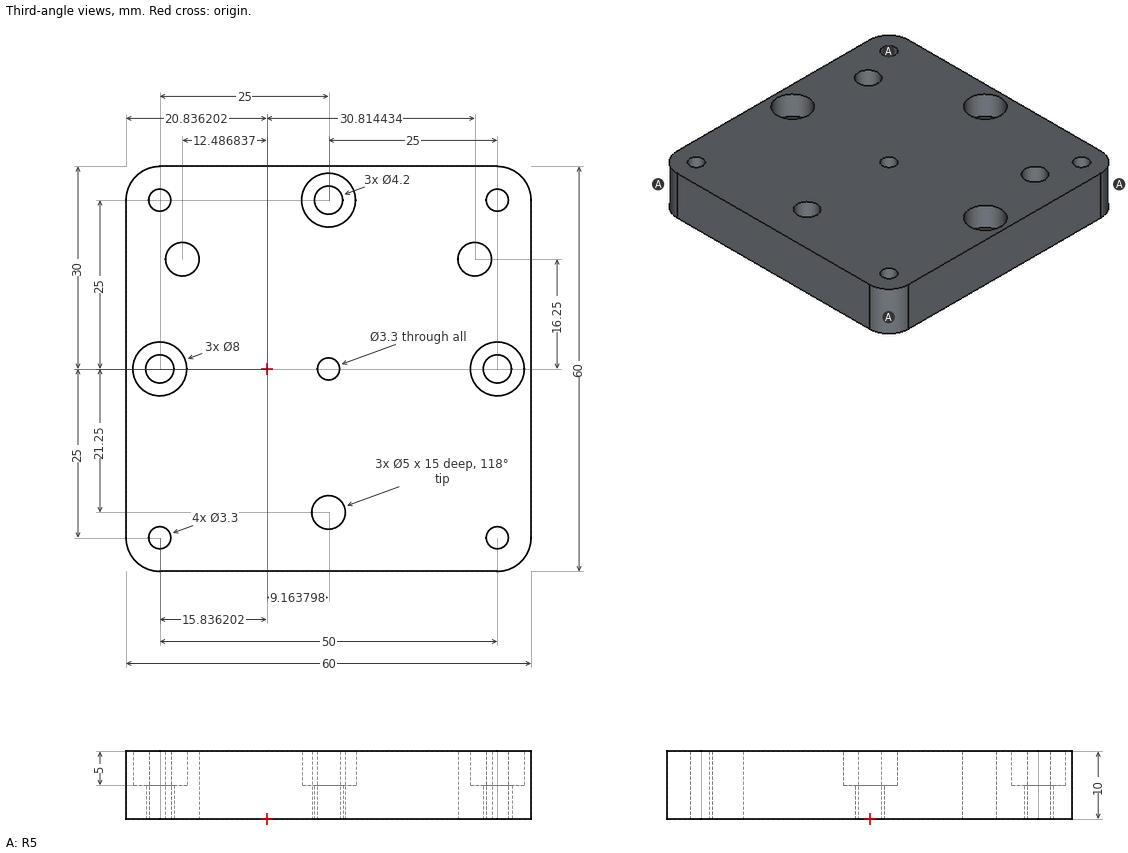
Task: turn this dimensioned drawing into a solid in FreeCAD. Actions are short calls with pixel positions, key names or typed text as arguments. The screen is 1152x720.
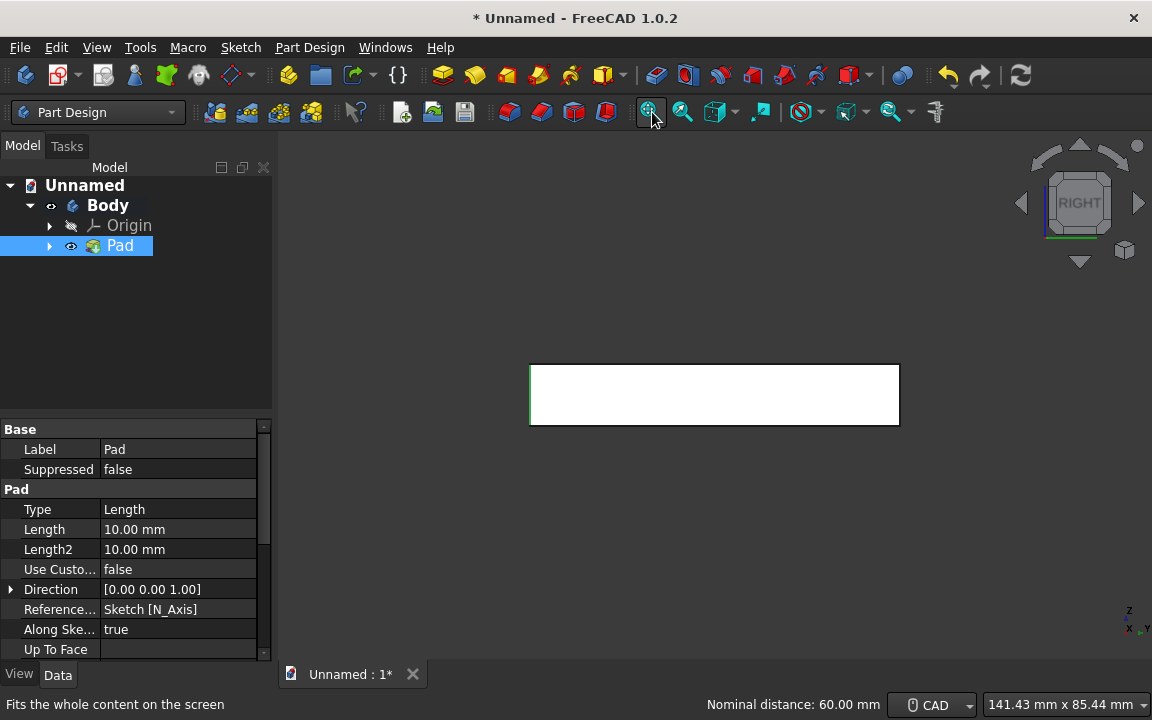
click(900, 394, ctrl)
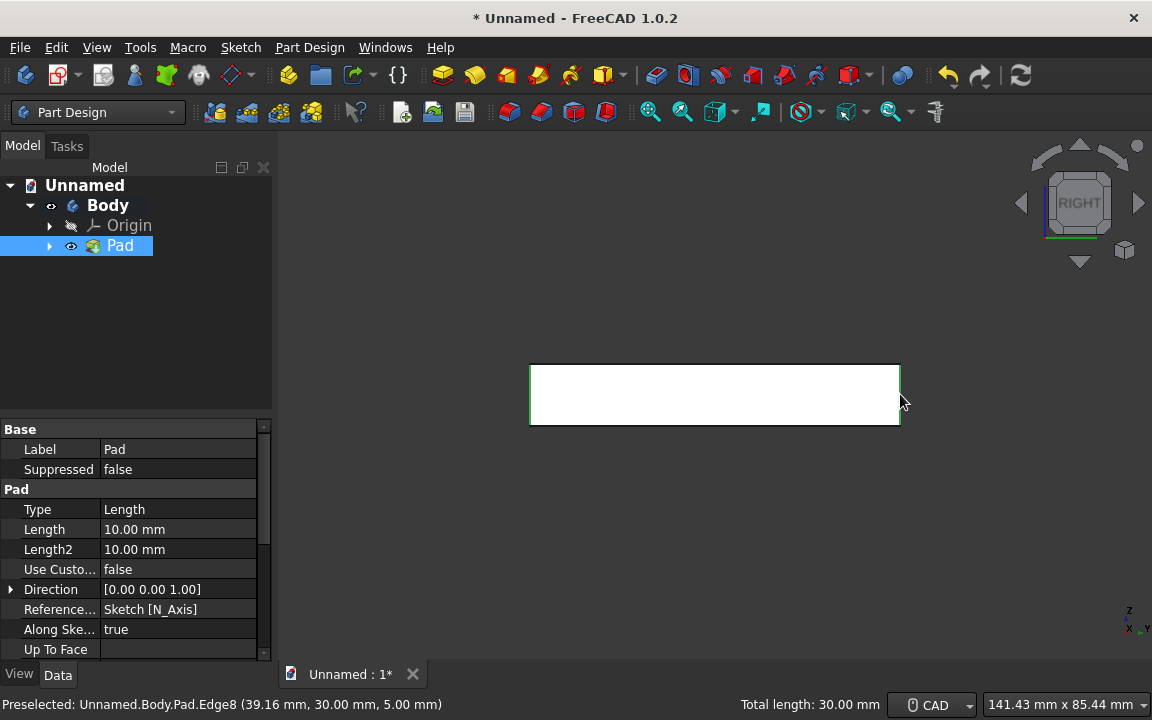
key(5)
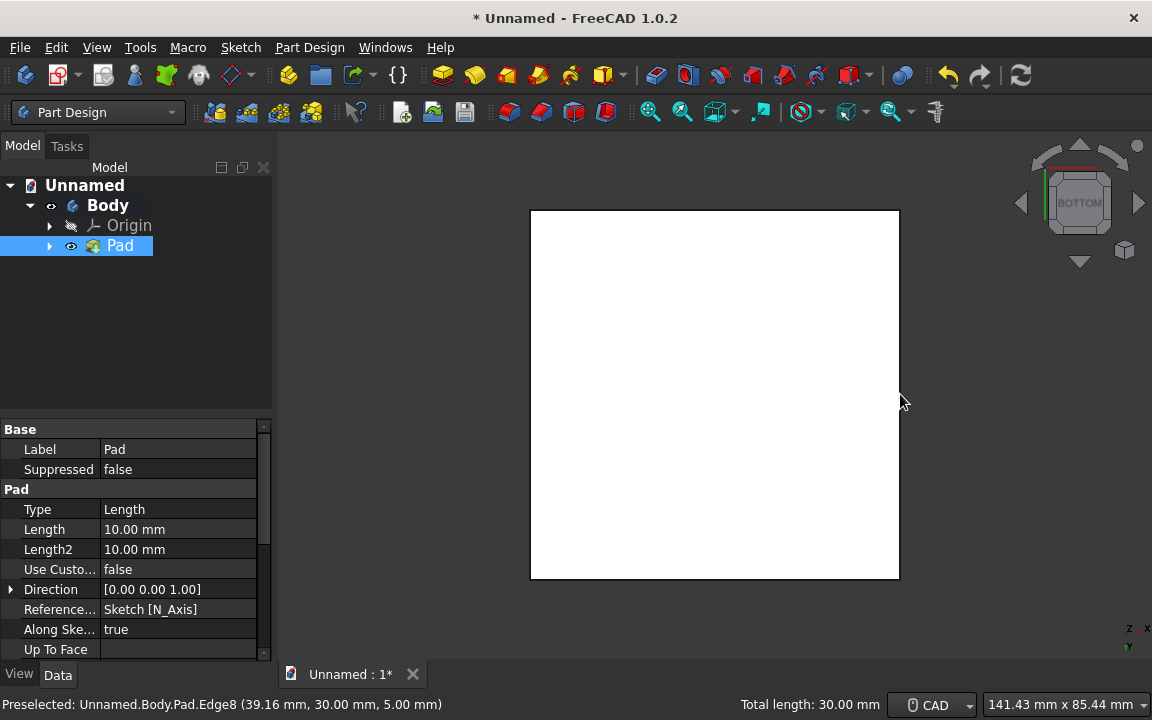
key(4)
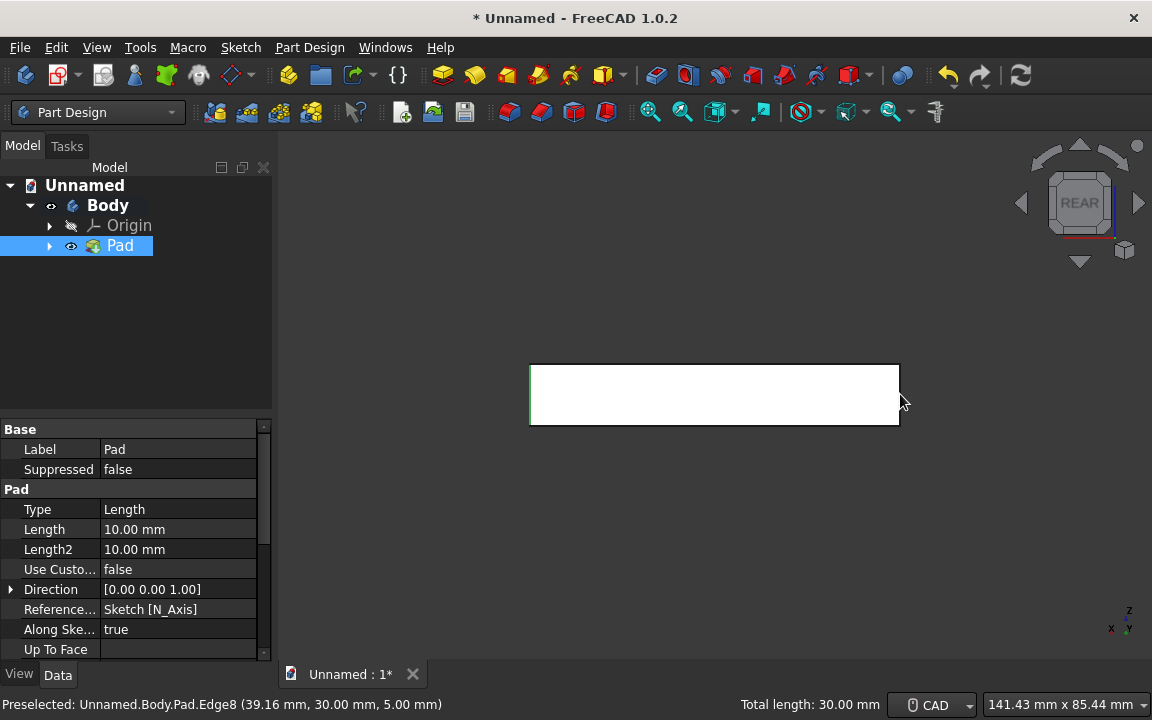
click(652, 112)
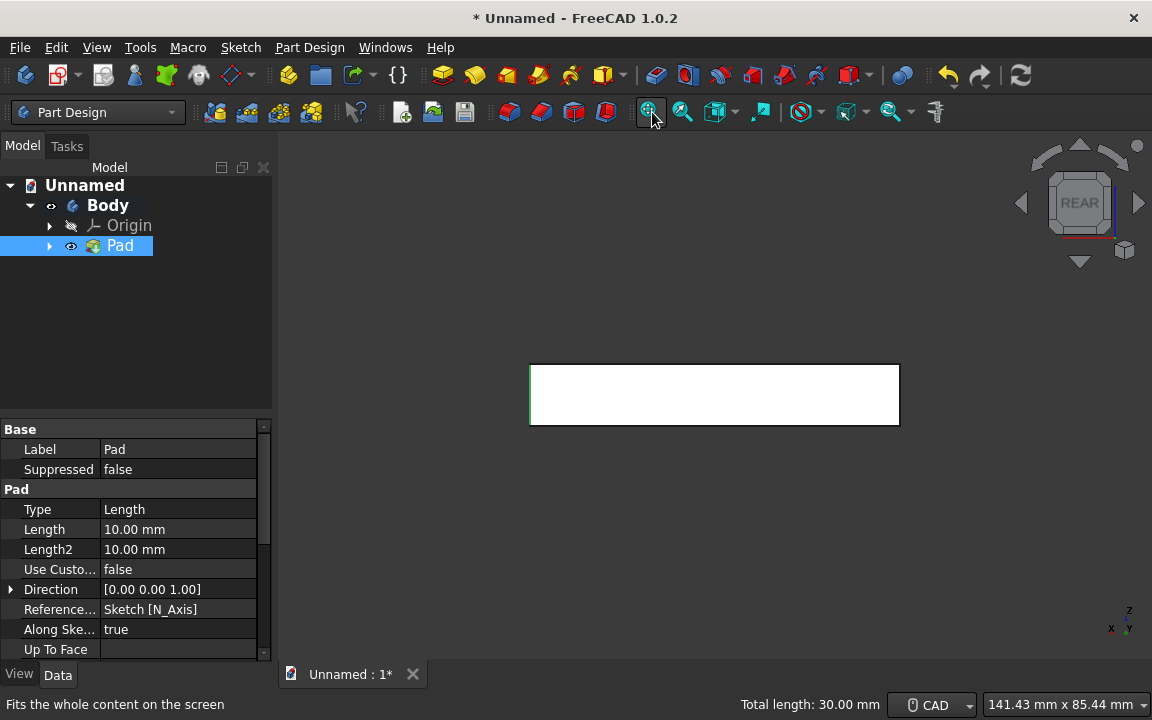
click(900, 394, ctrl)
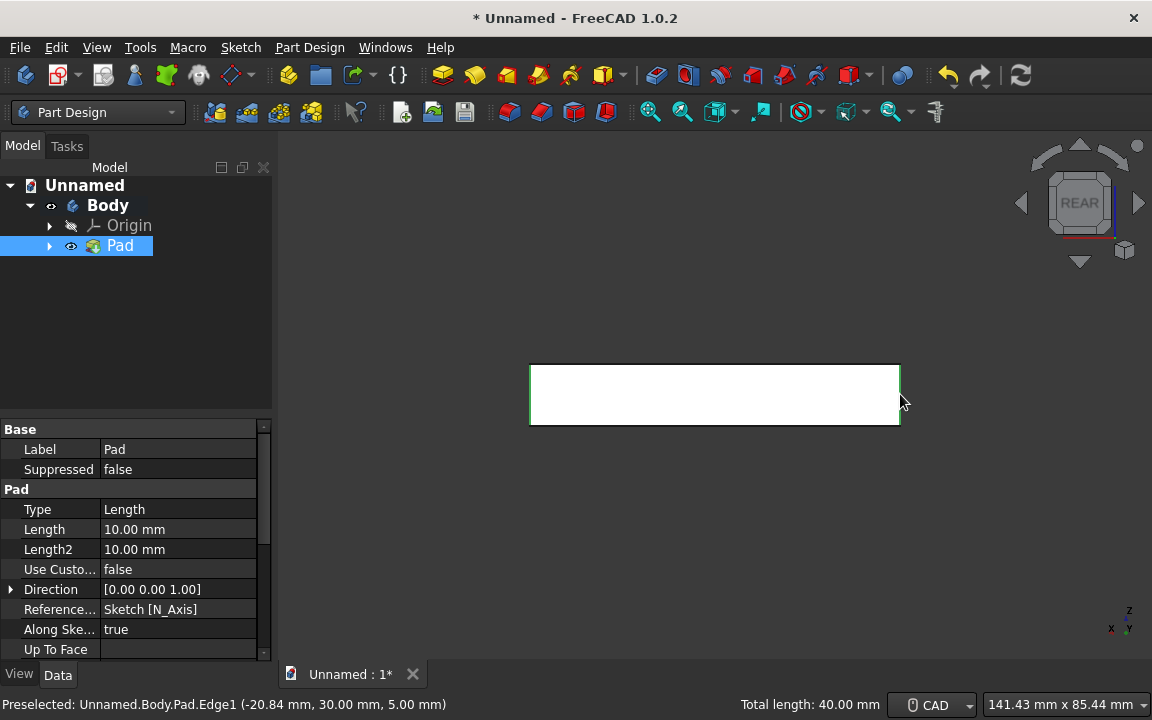
click(510, 112)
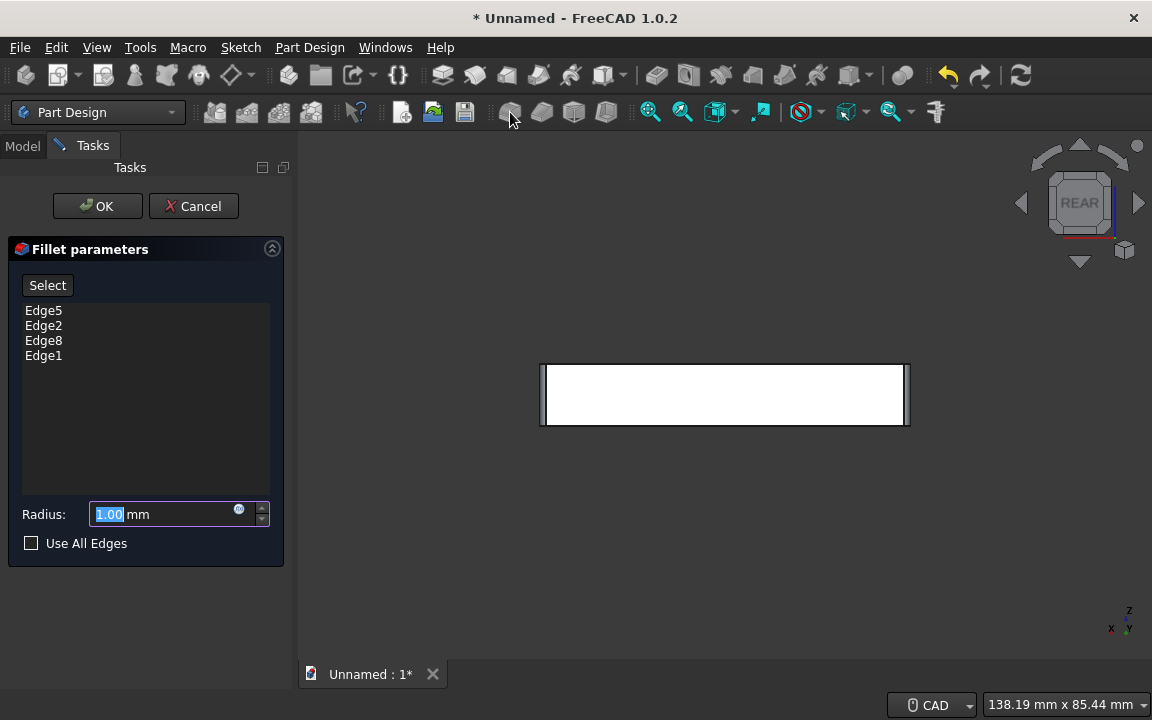
text(5)
key(Tab)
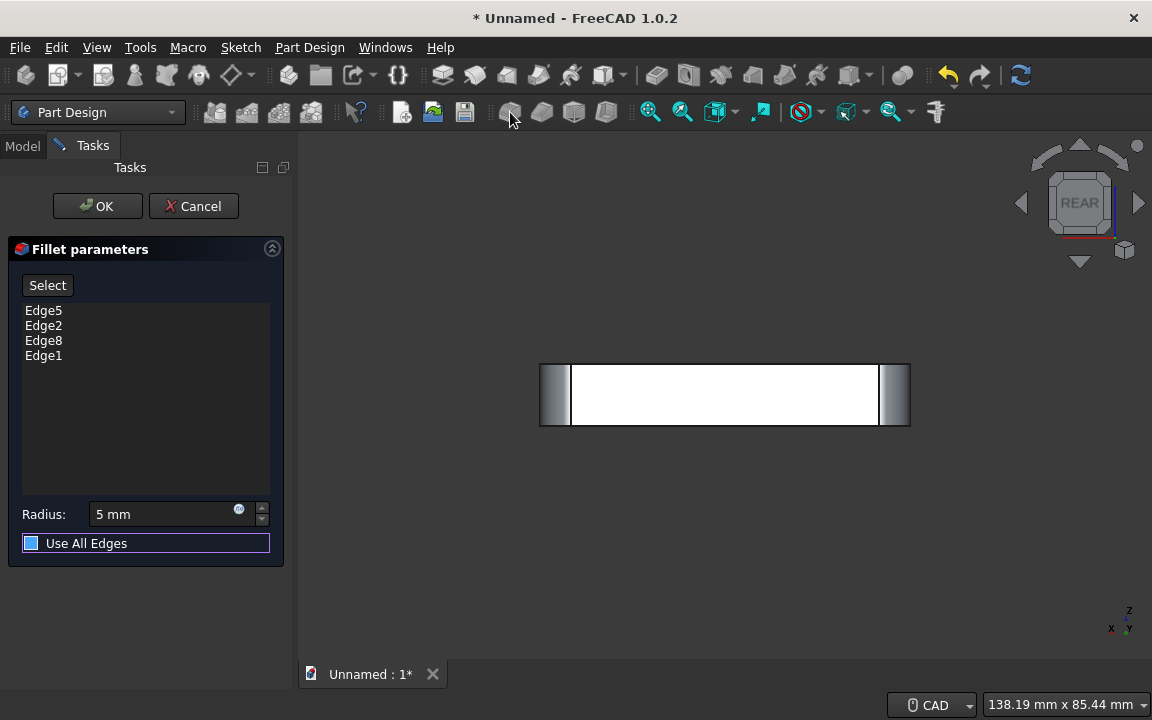
click(98, 206)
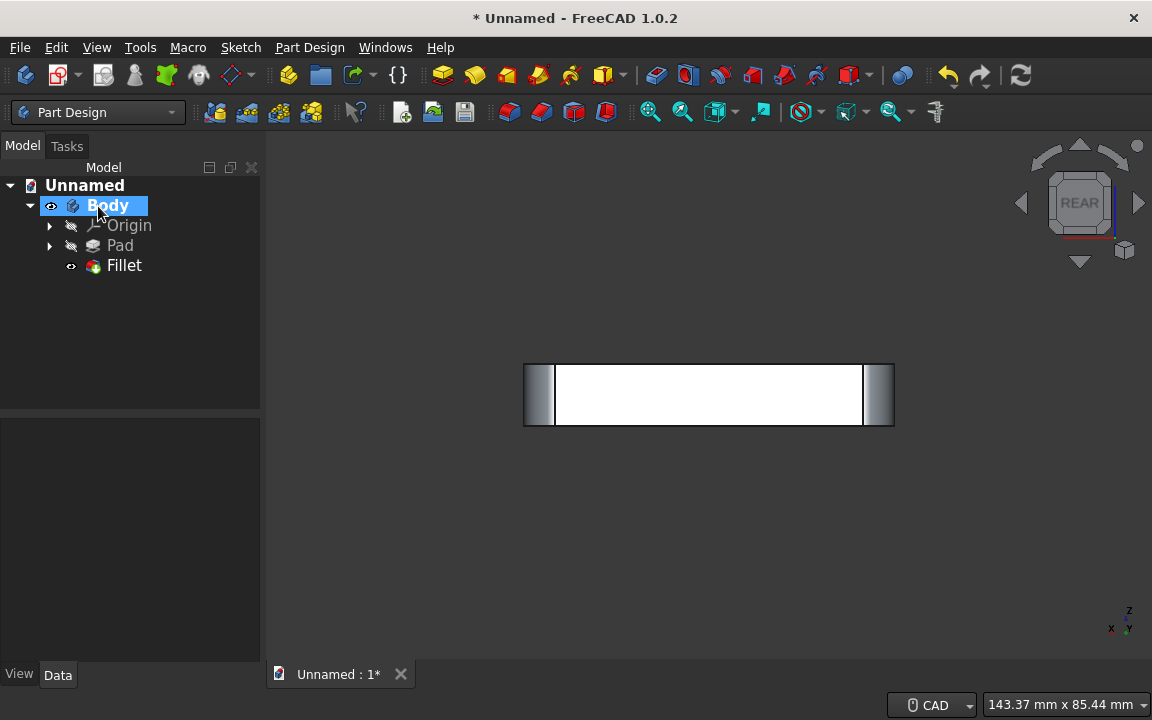
click(652, 112)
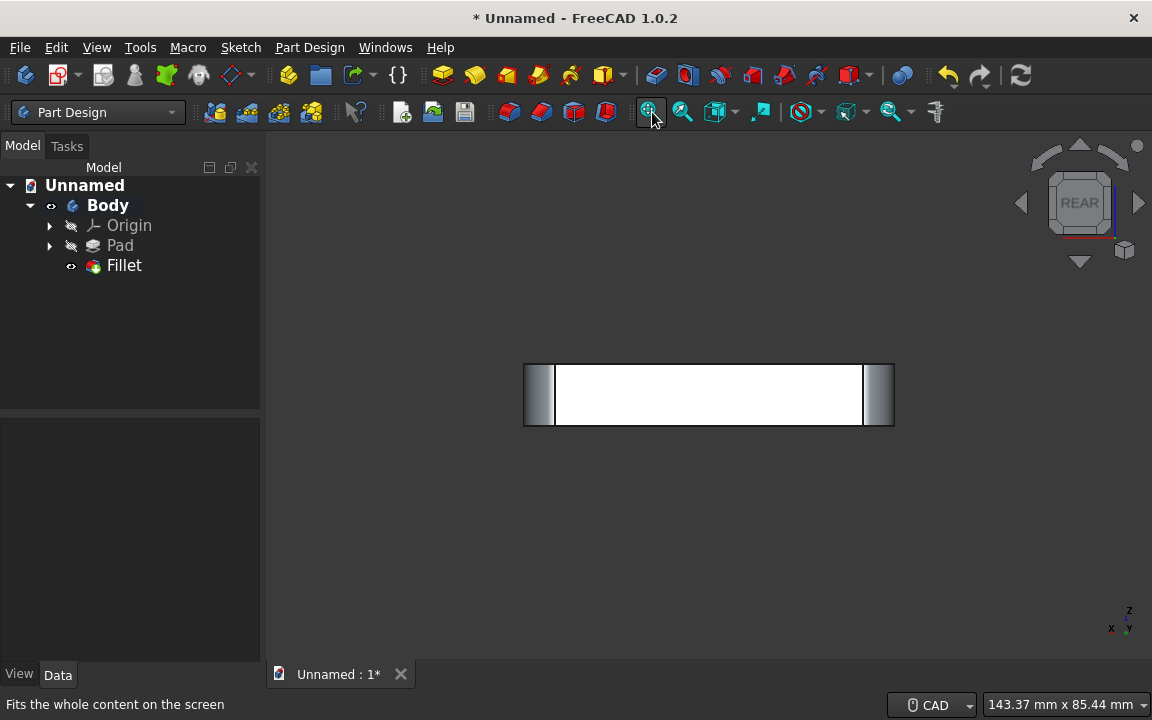
key(0)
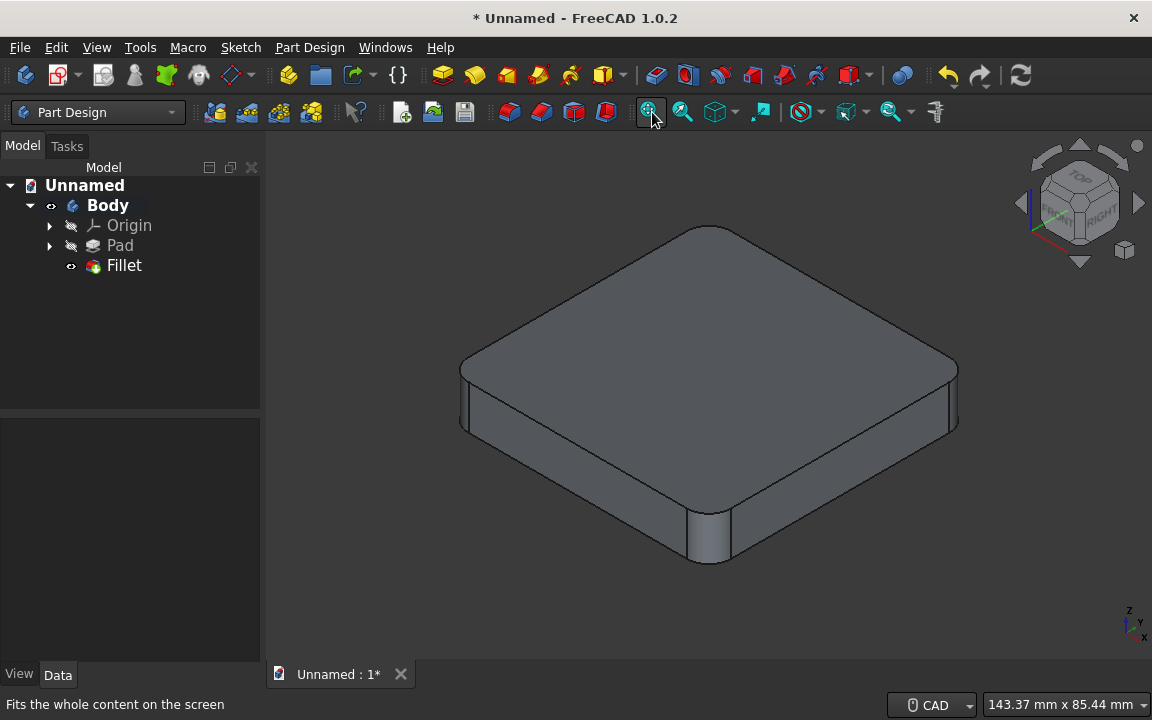
click(709, 369)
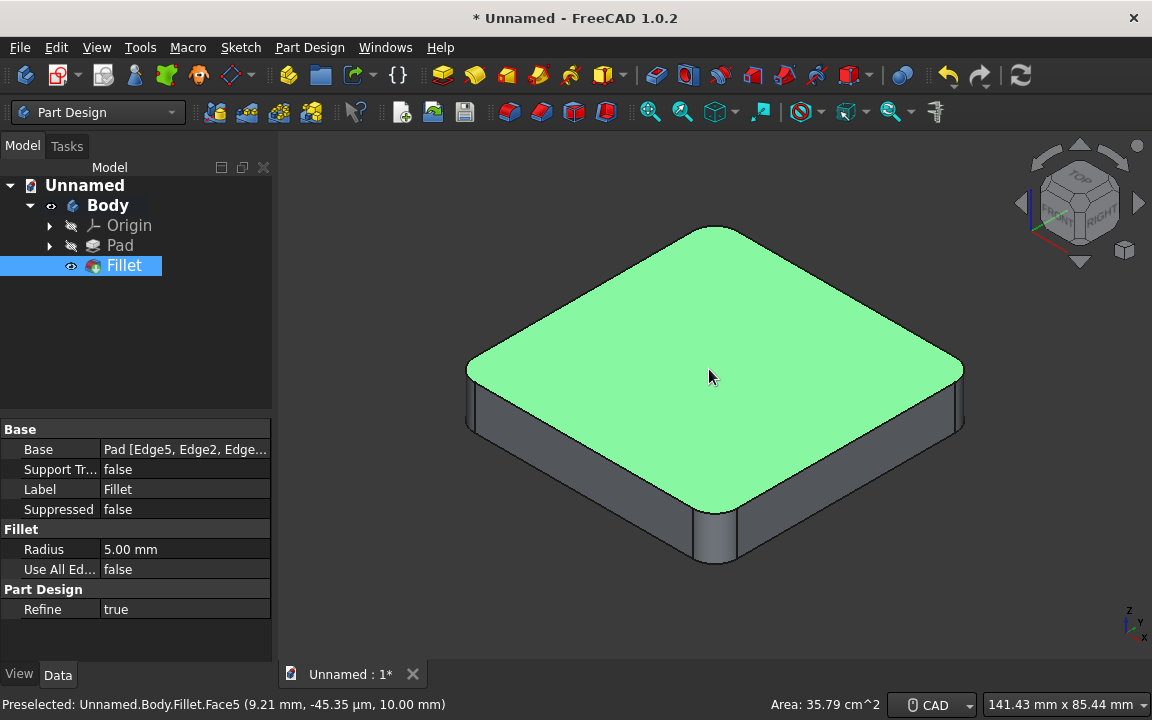
click(58, 76)